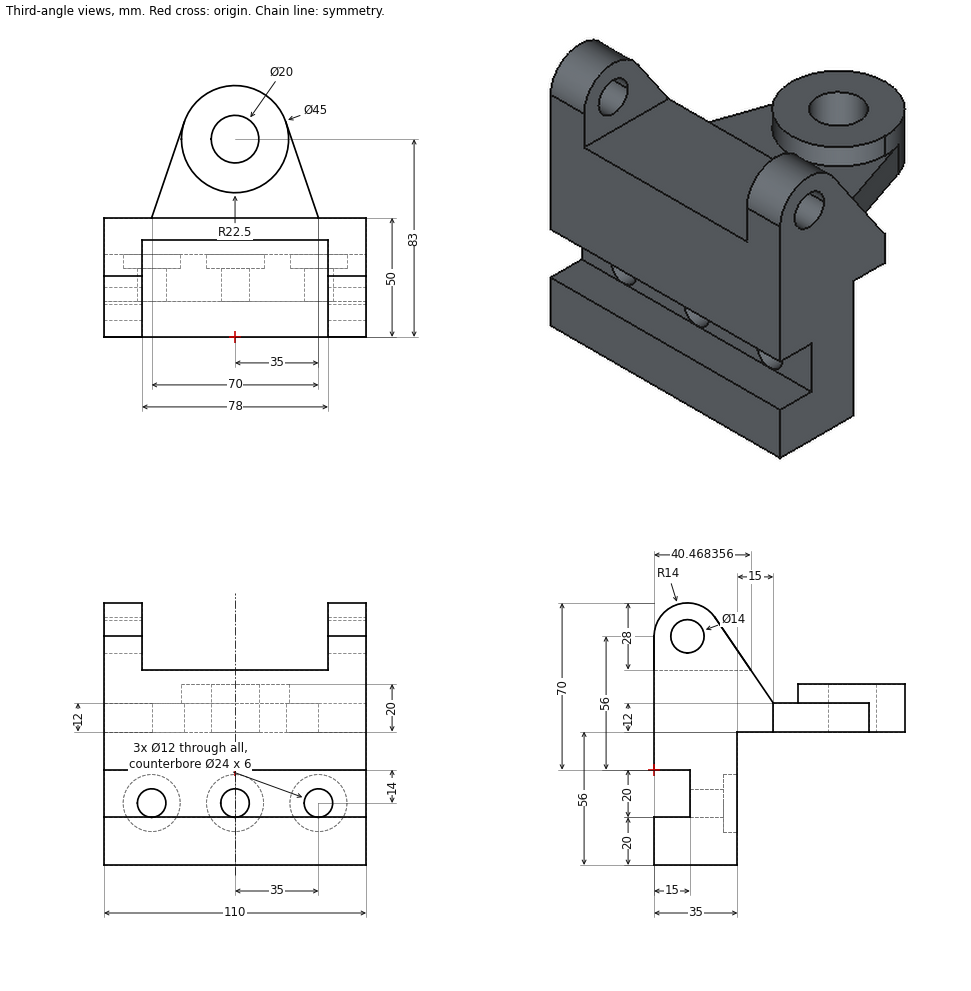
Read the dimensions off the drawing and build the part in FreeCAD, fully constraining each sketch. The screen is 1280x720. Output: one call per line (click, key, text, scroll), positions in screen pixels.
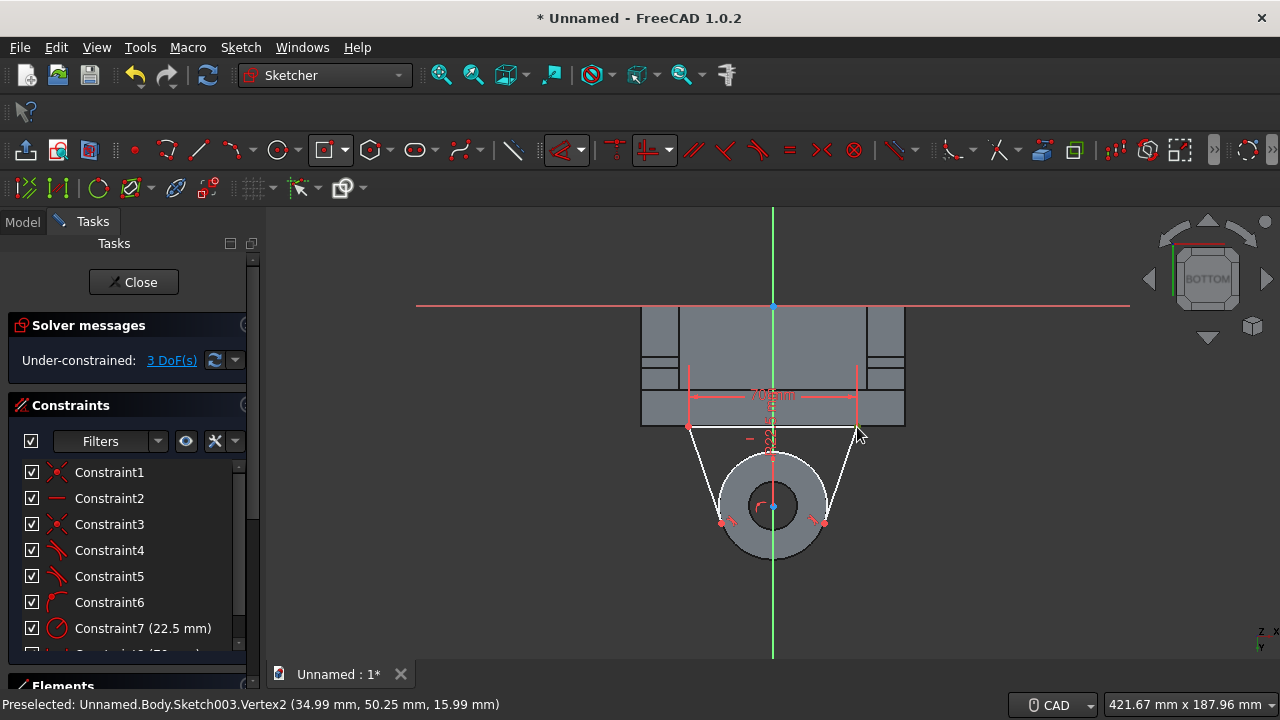
key(l)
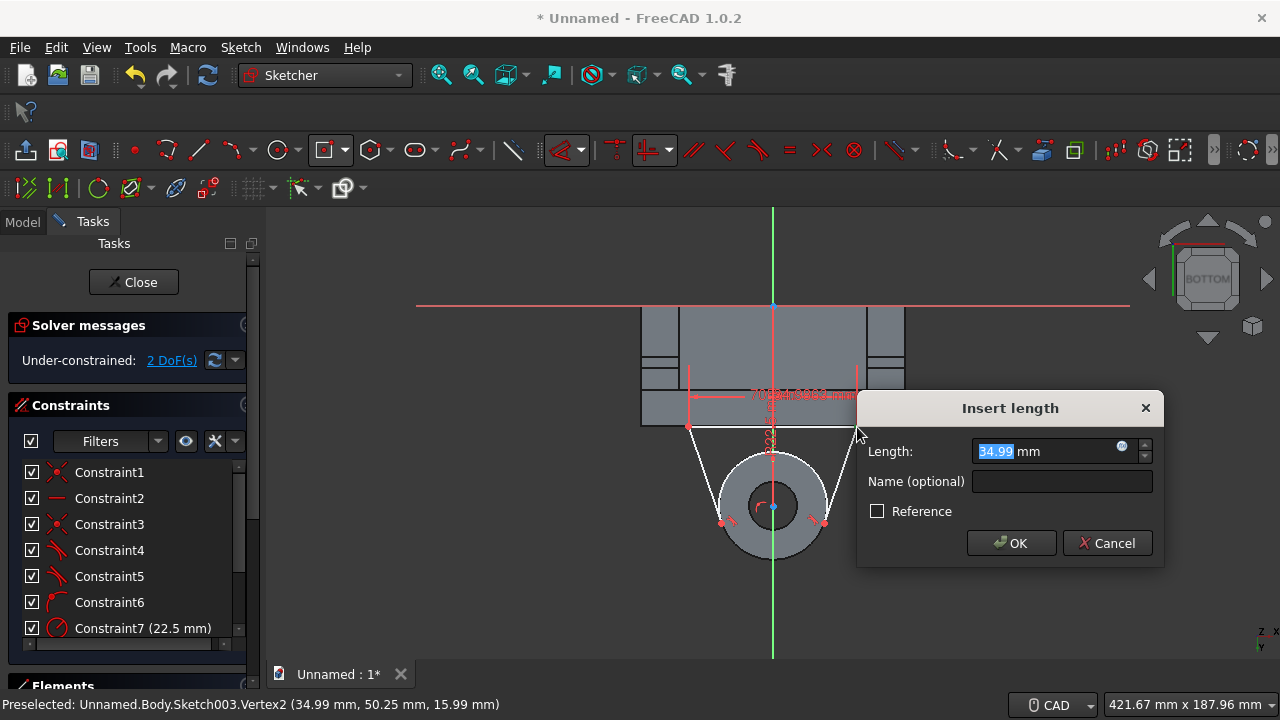
text(35)
key(Return)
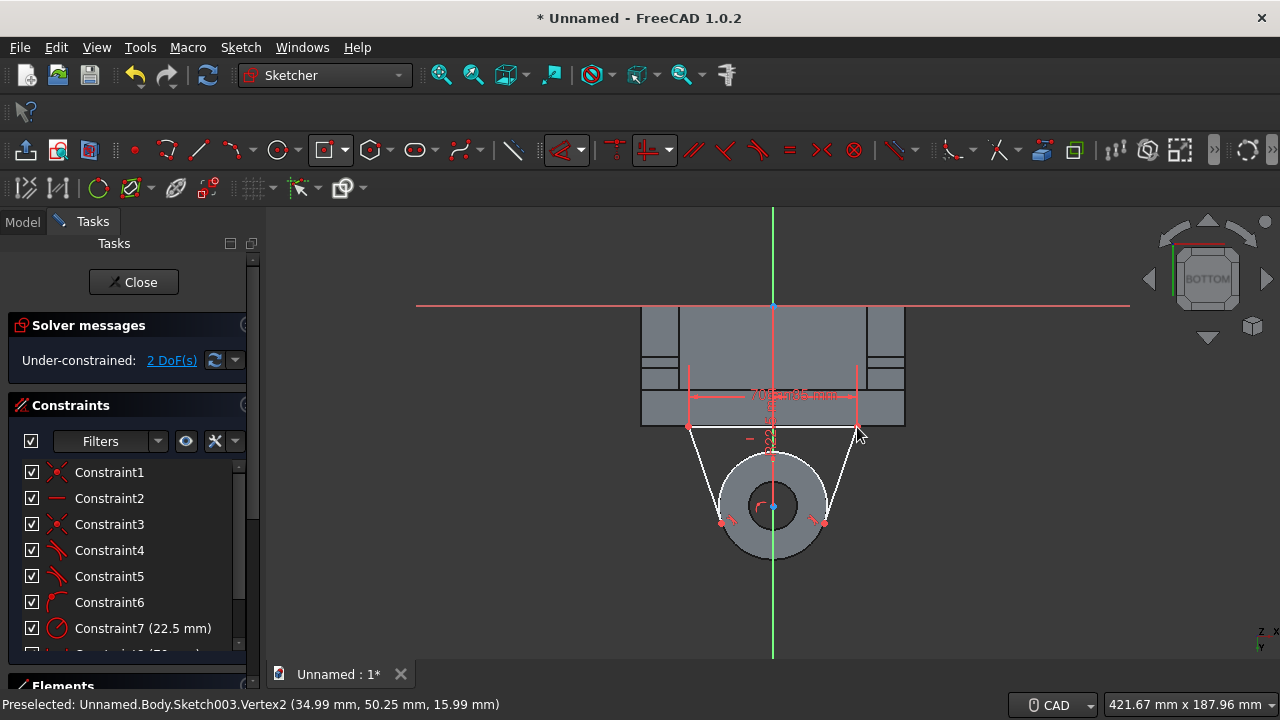
click(857, 427)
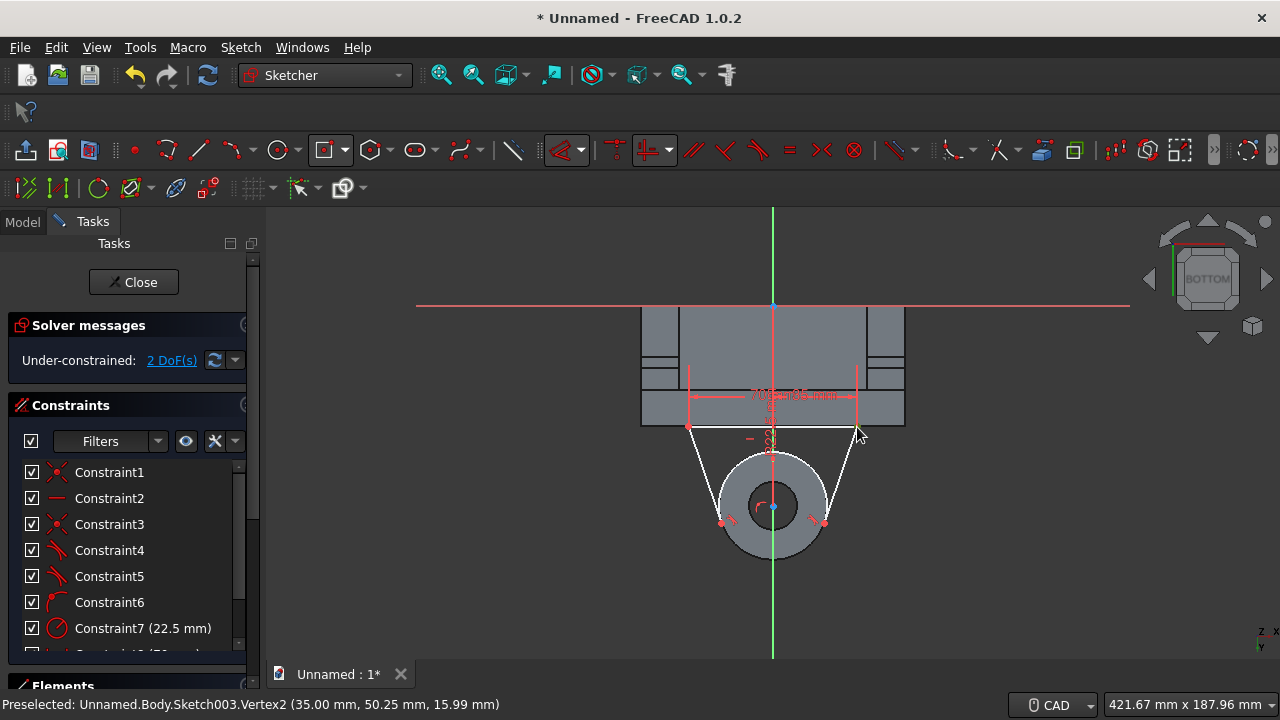
key(i)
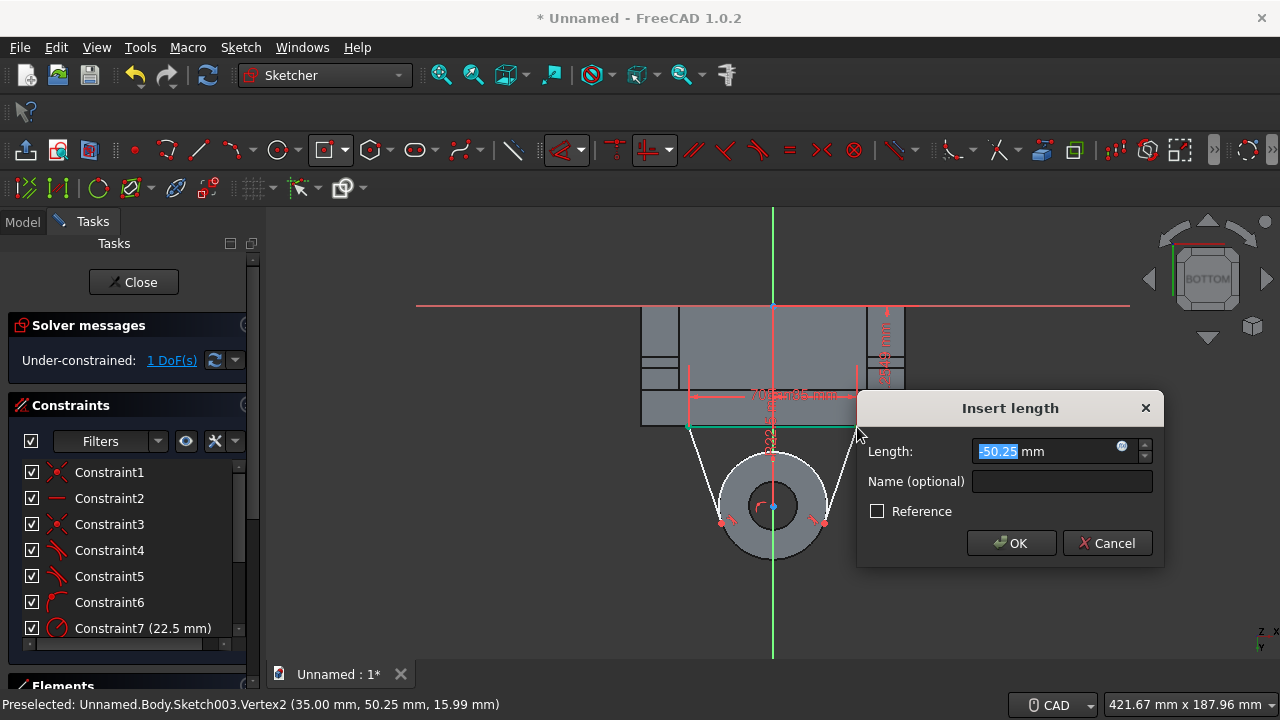
text(-50)
key(Return)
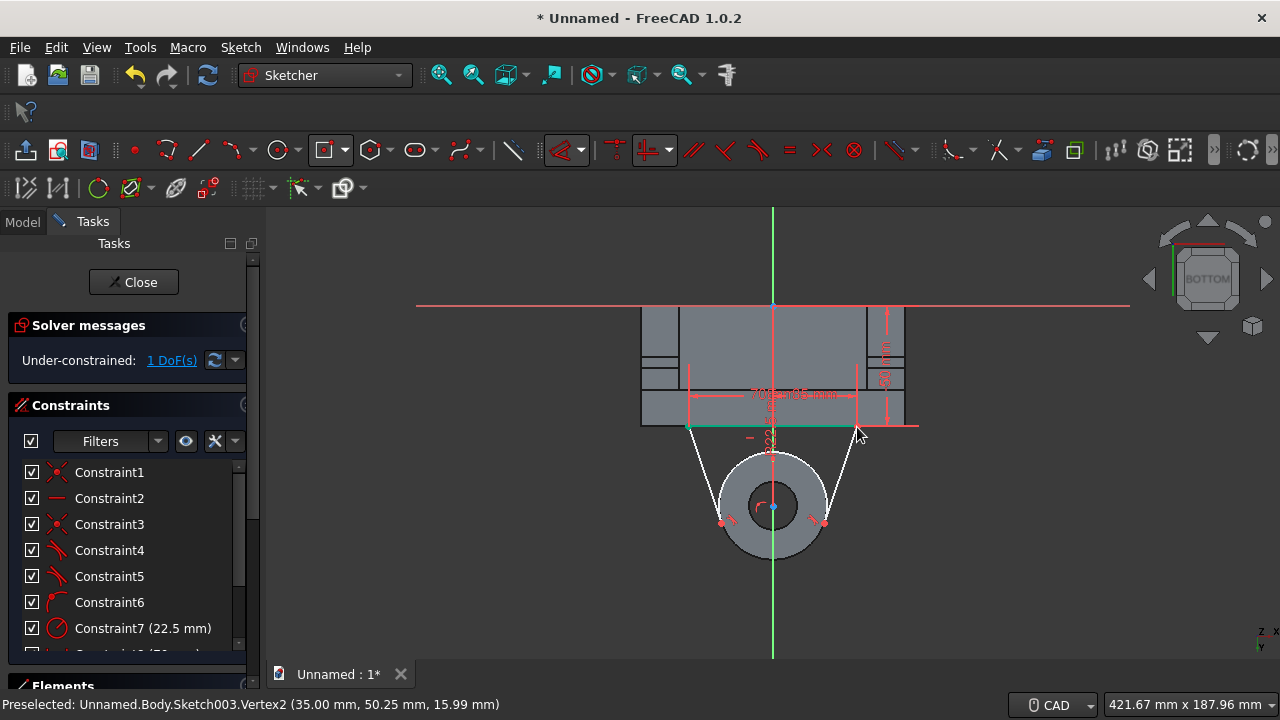
click(773, 506)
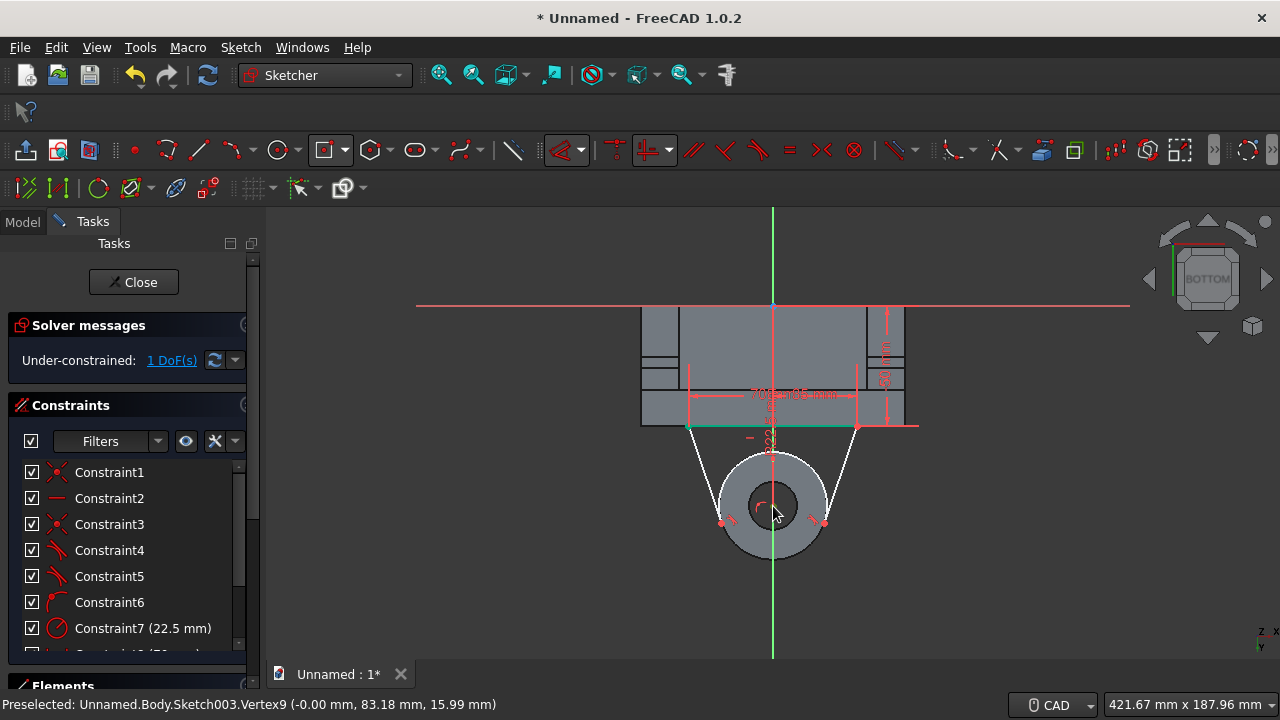
click(584, 150)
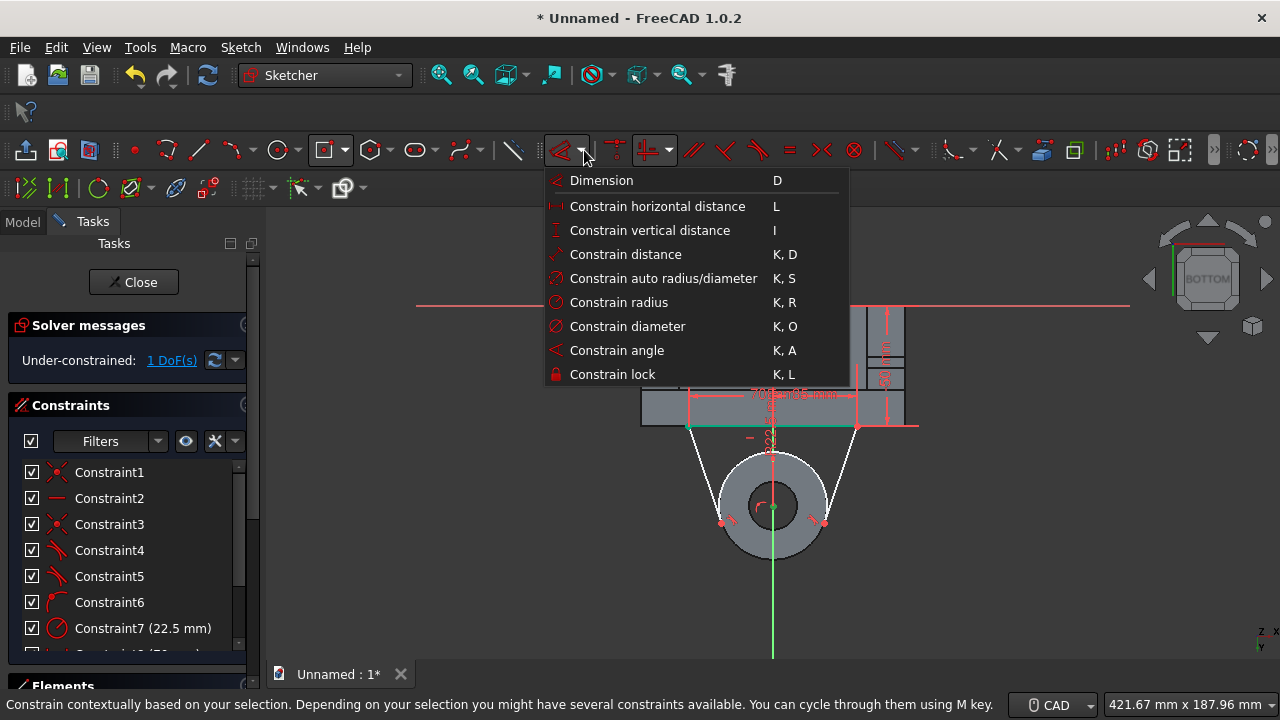
click(697, 230)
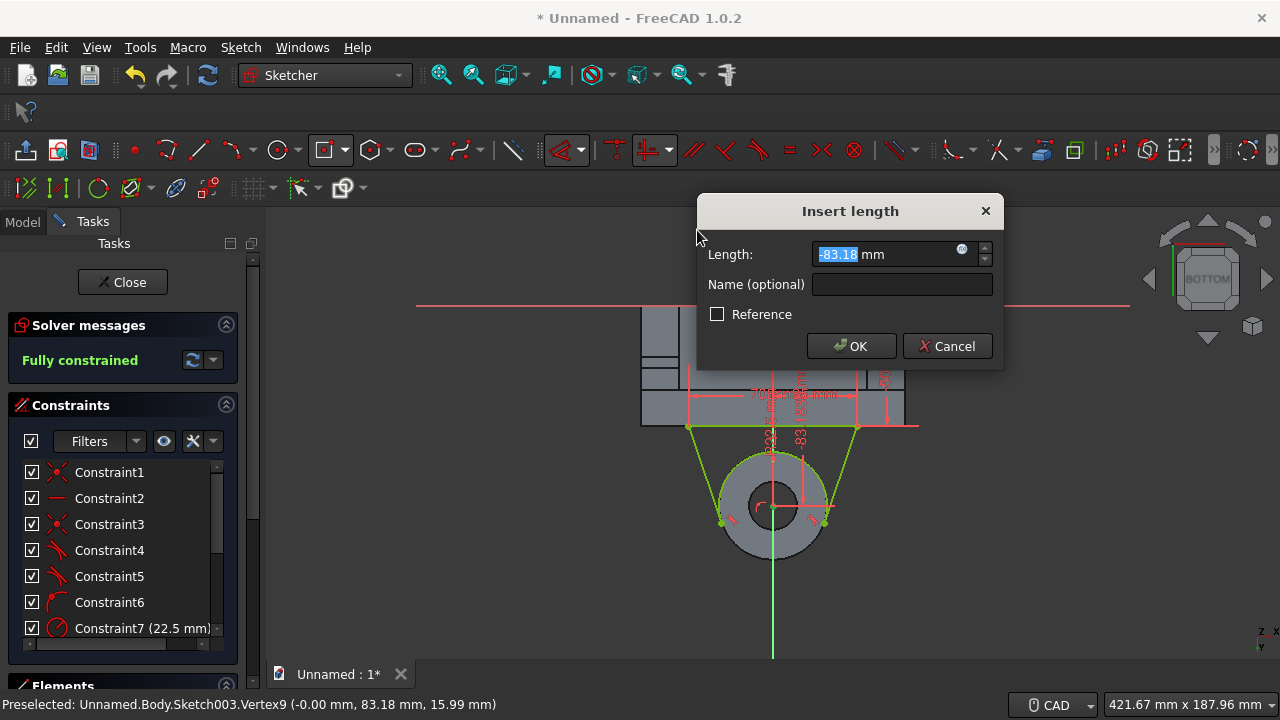
text(-83)
key(Return)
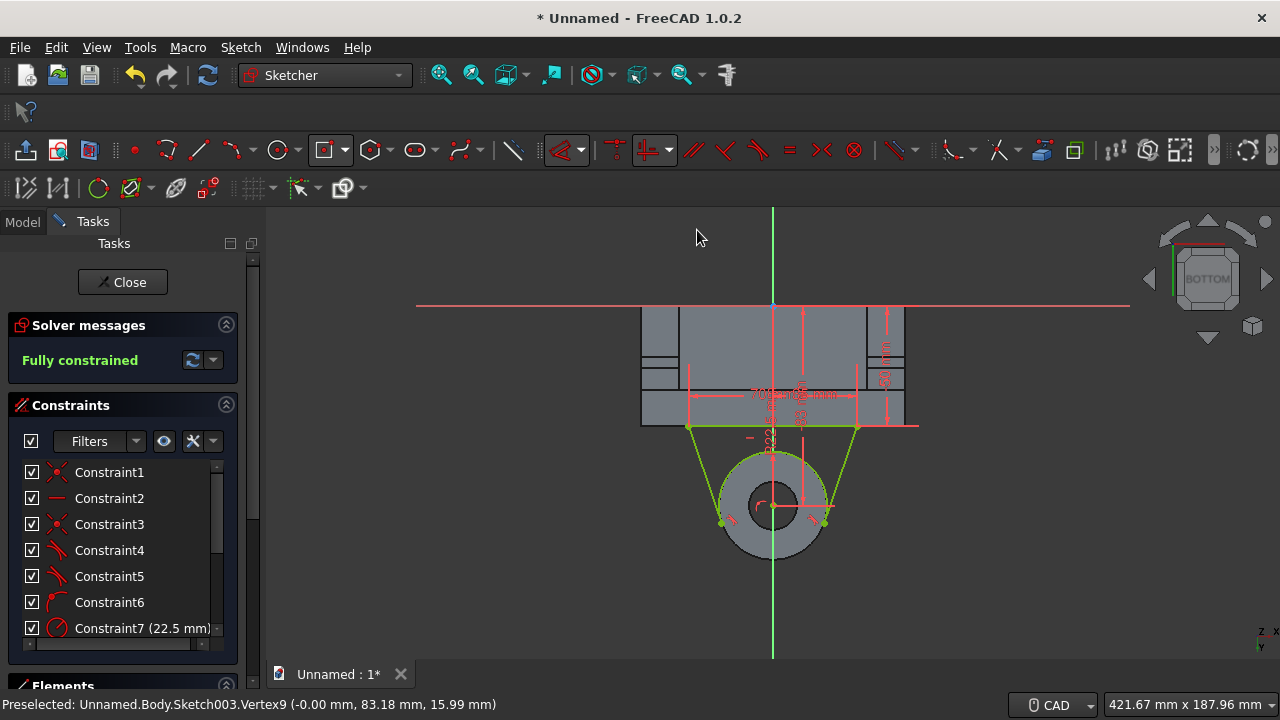
click(123, 282)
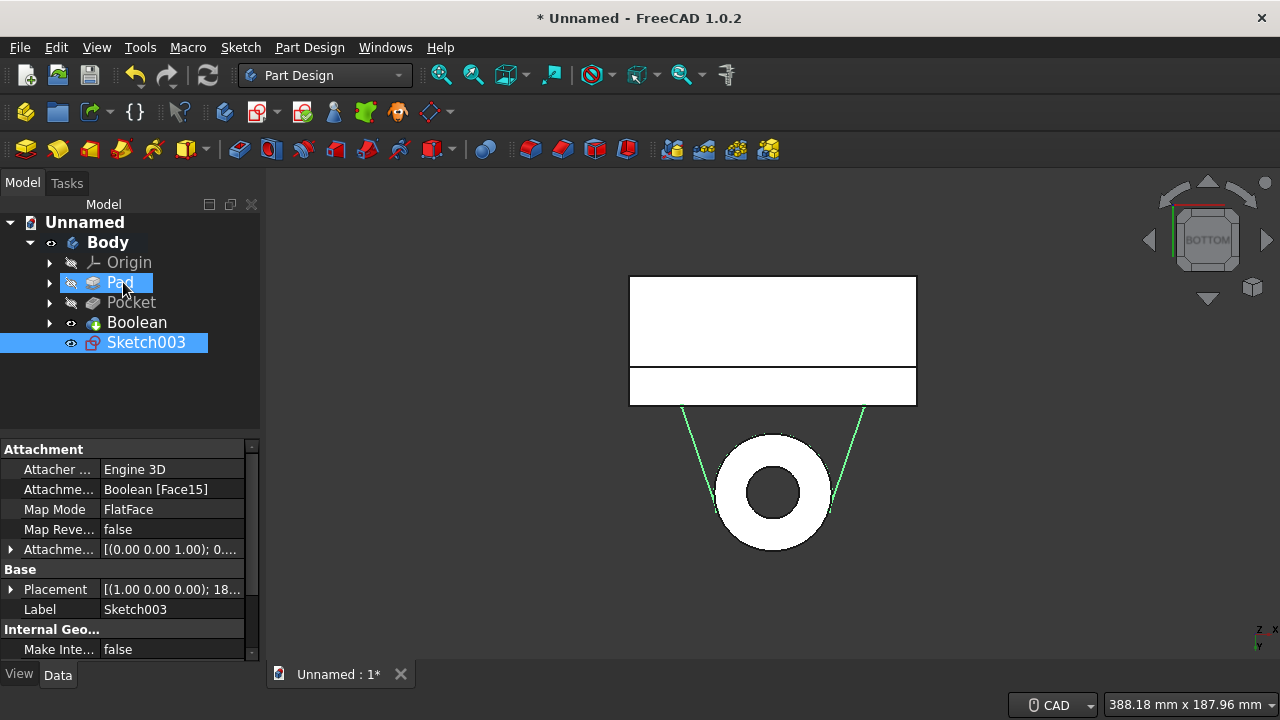
click(26, 150)